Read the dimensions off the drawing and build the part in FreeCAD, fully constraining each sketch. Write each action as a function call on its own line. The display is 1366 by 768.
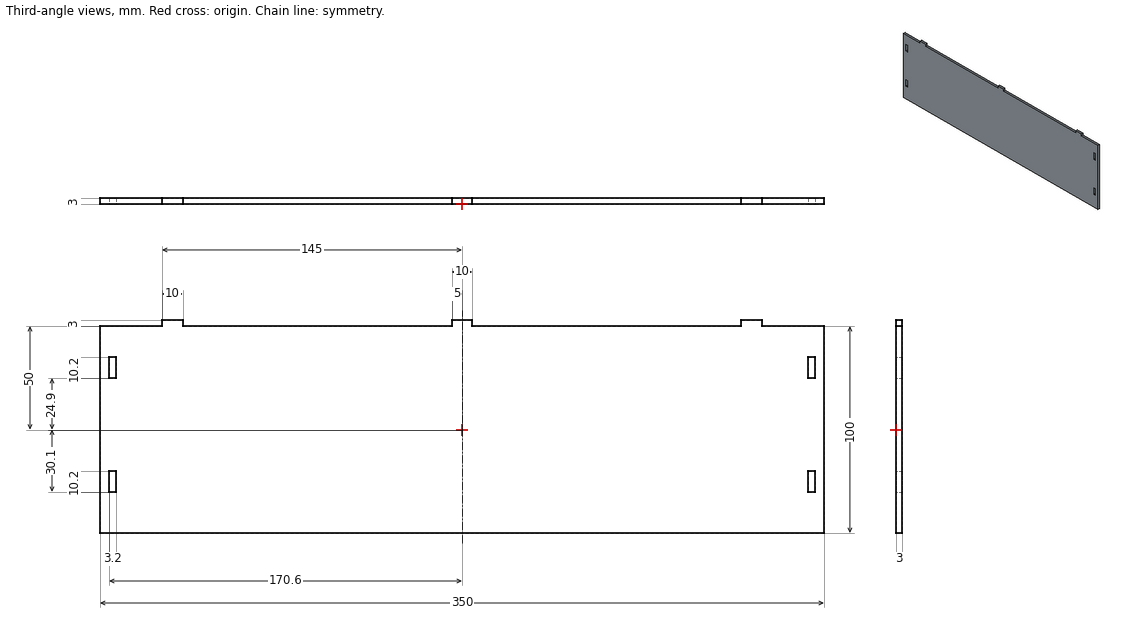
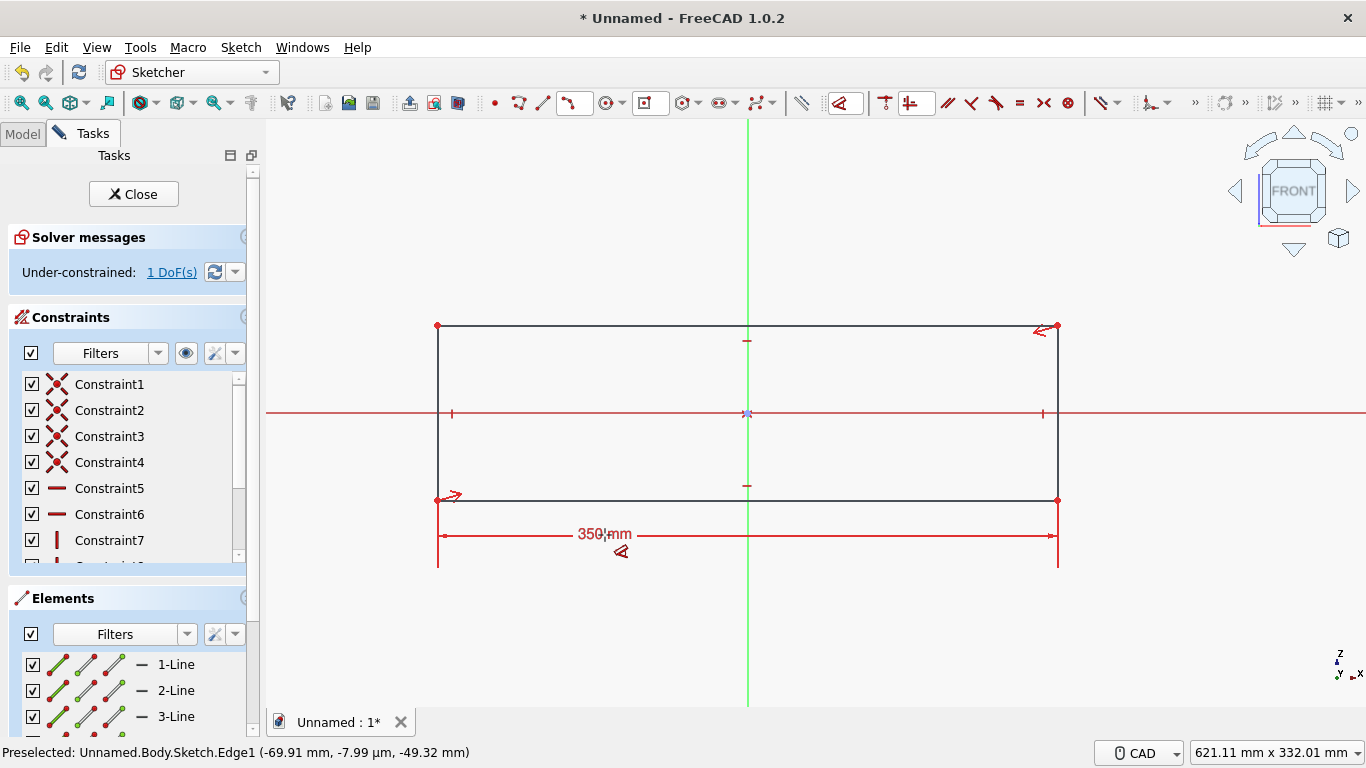
click(1058, 448)
click(1092, 373)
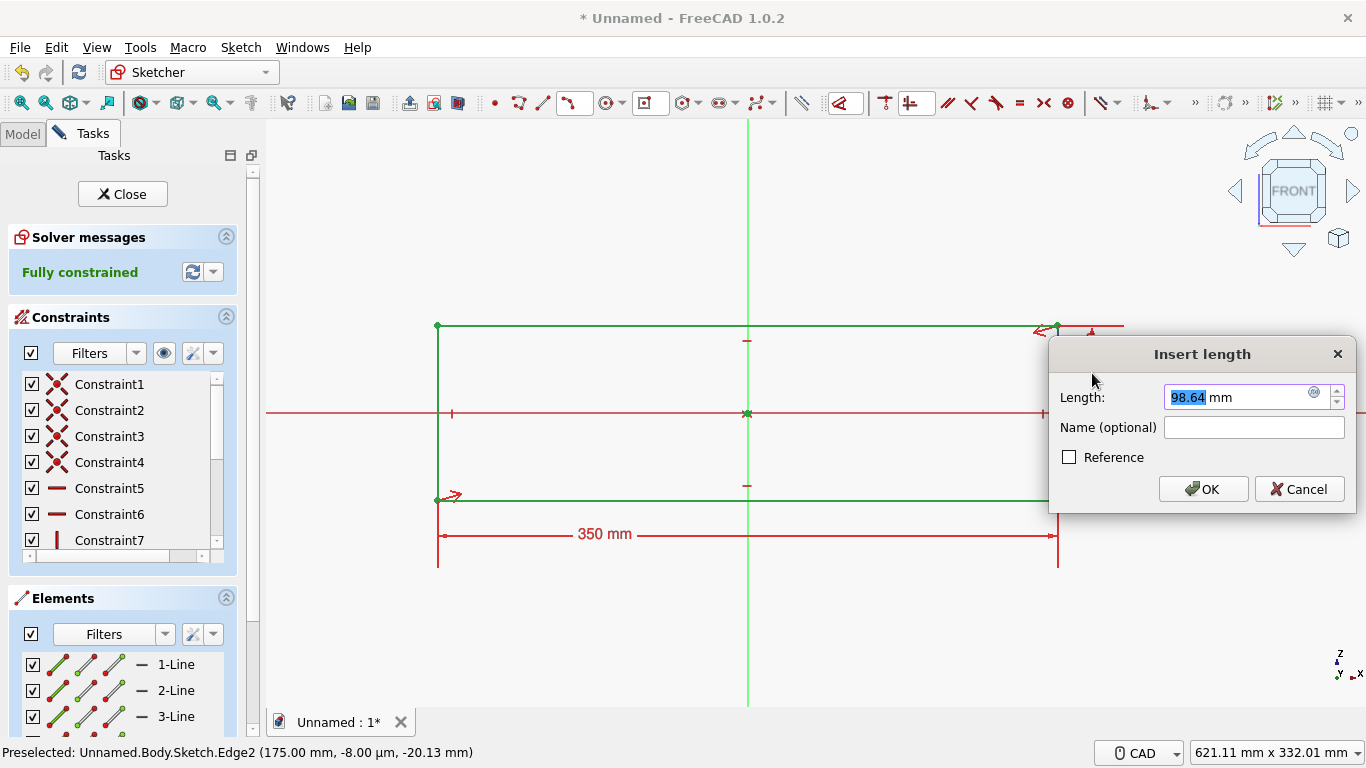
text(100)
key(Return)
key(Escape)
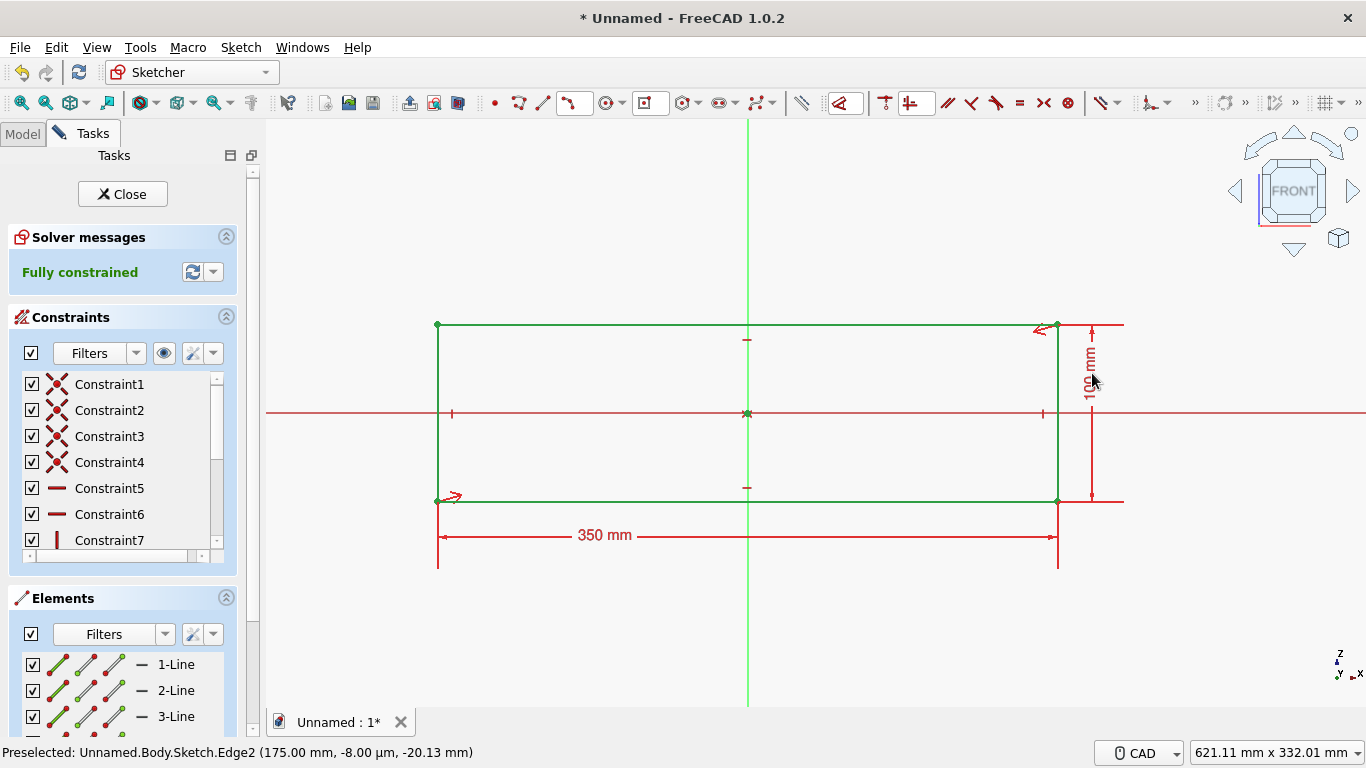
click(123, 194)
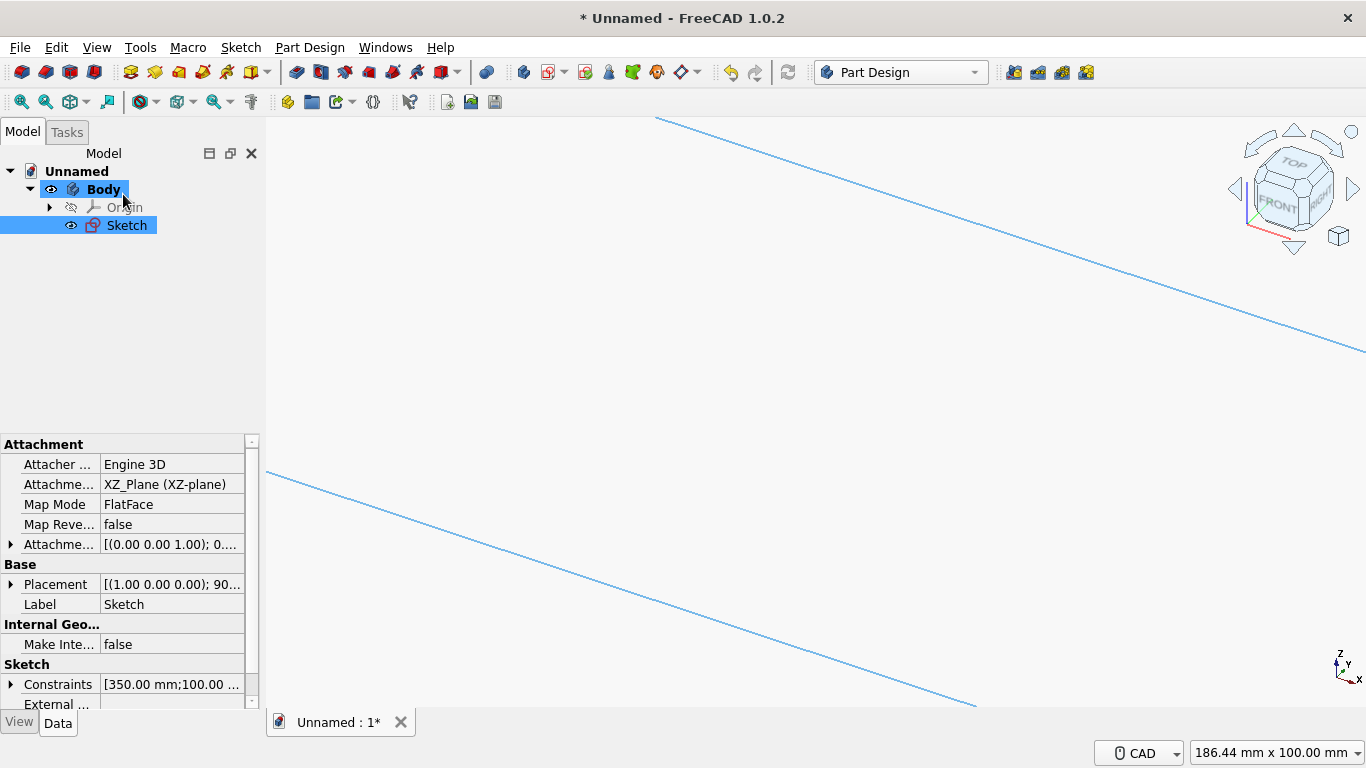
click(132, 72)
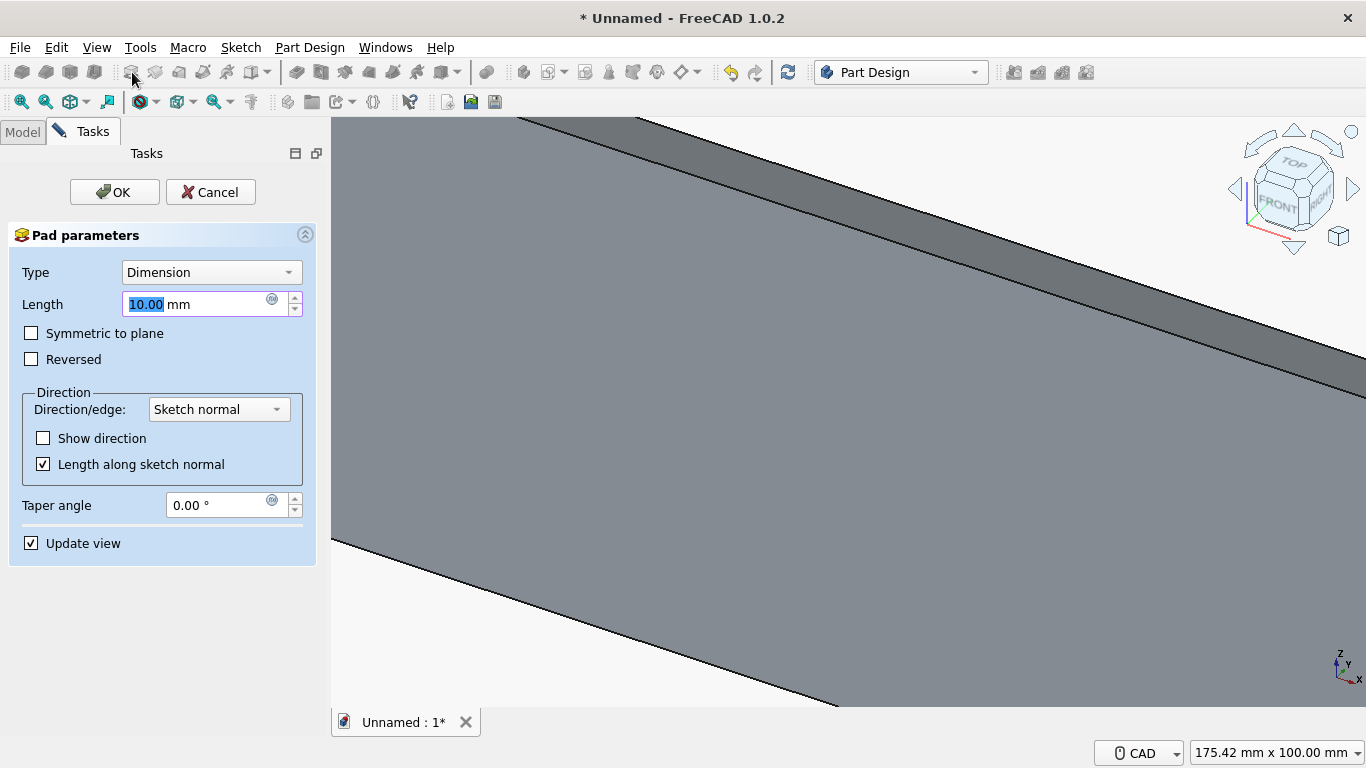
text(3)
key(Tab)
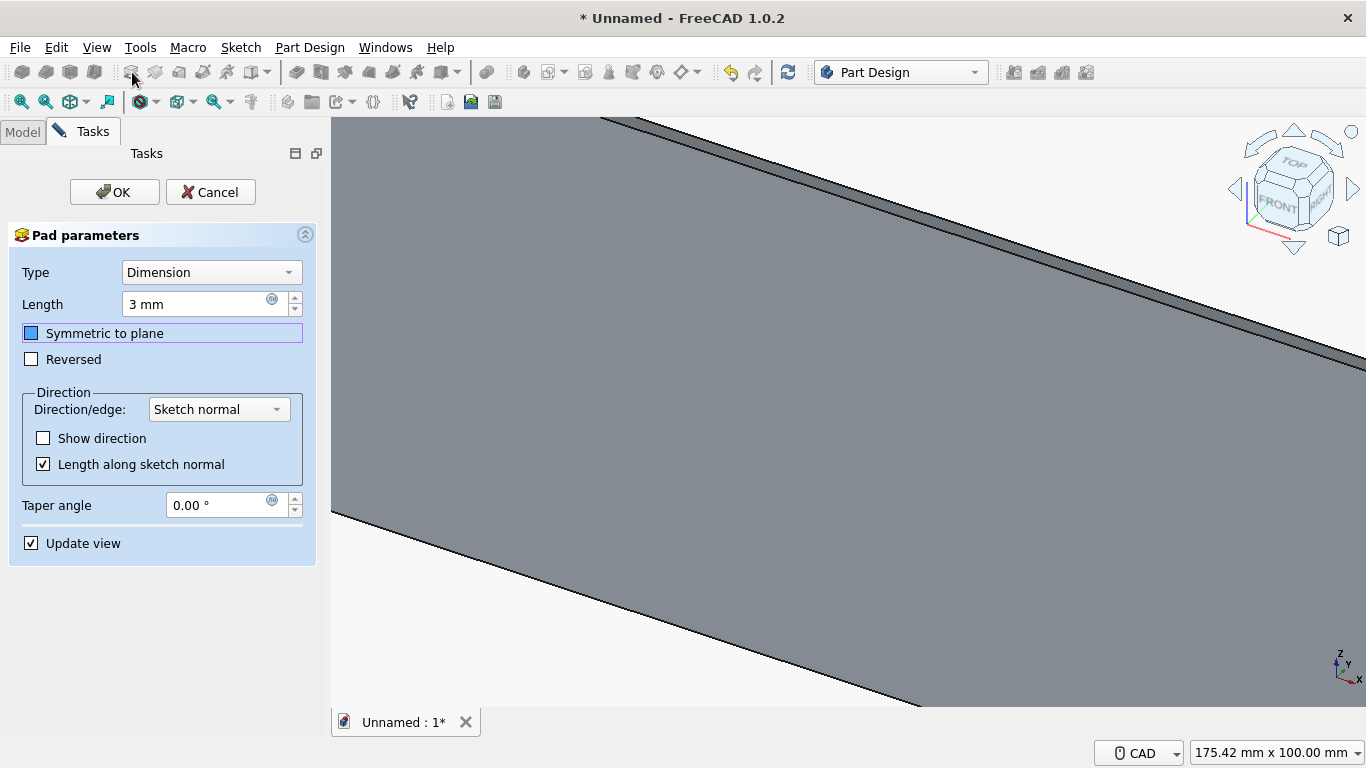
click(30, 359)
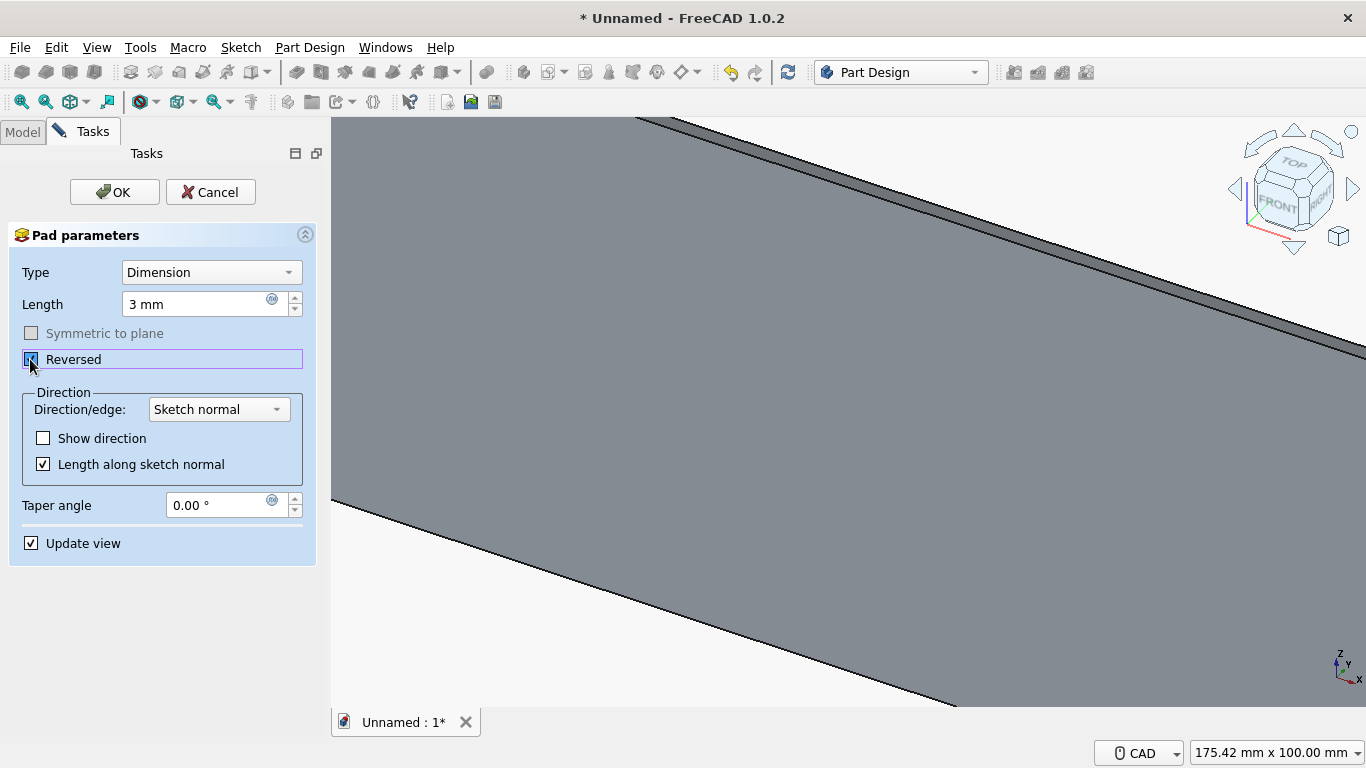
click(115, 192)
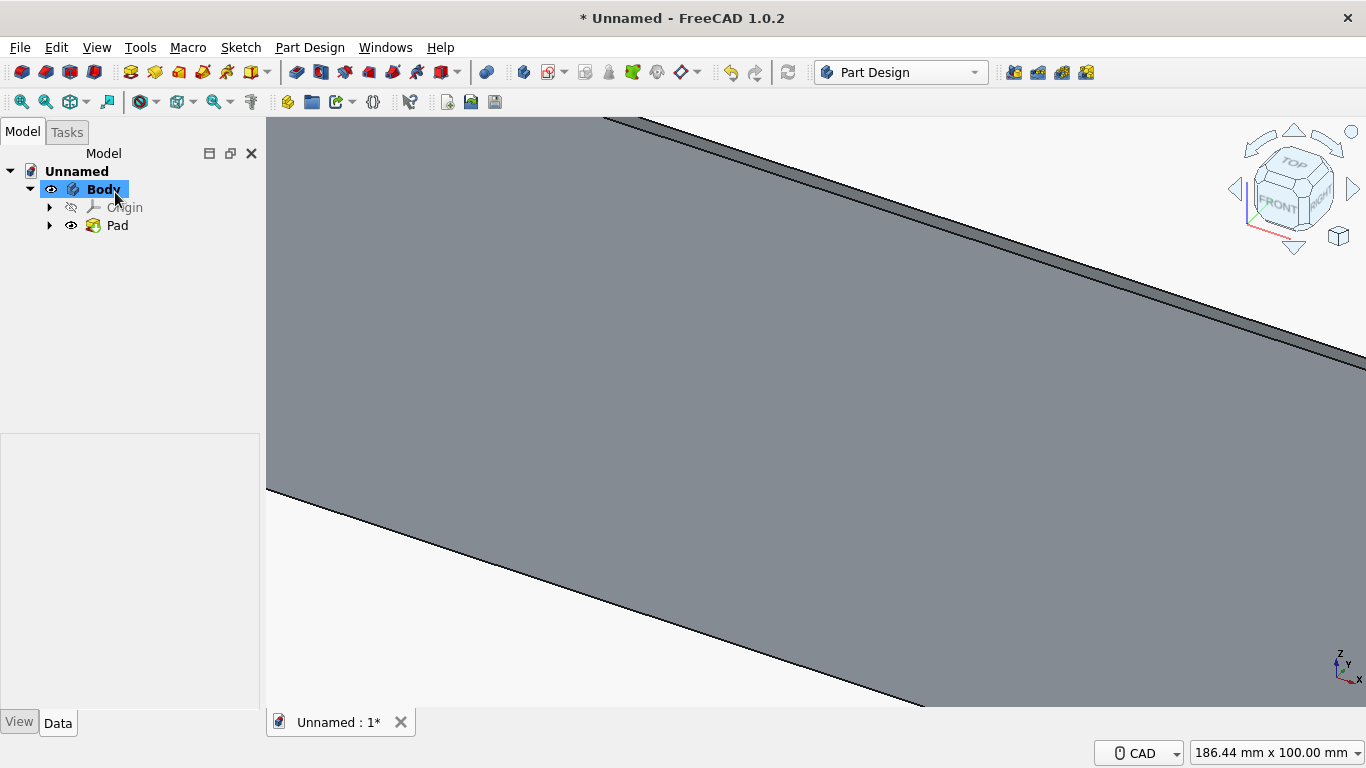
key(v)
key(f)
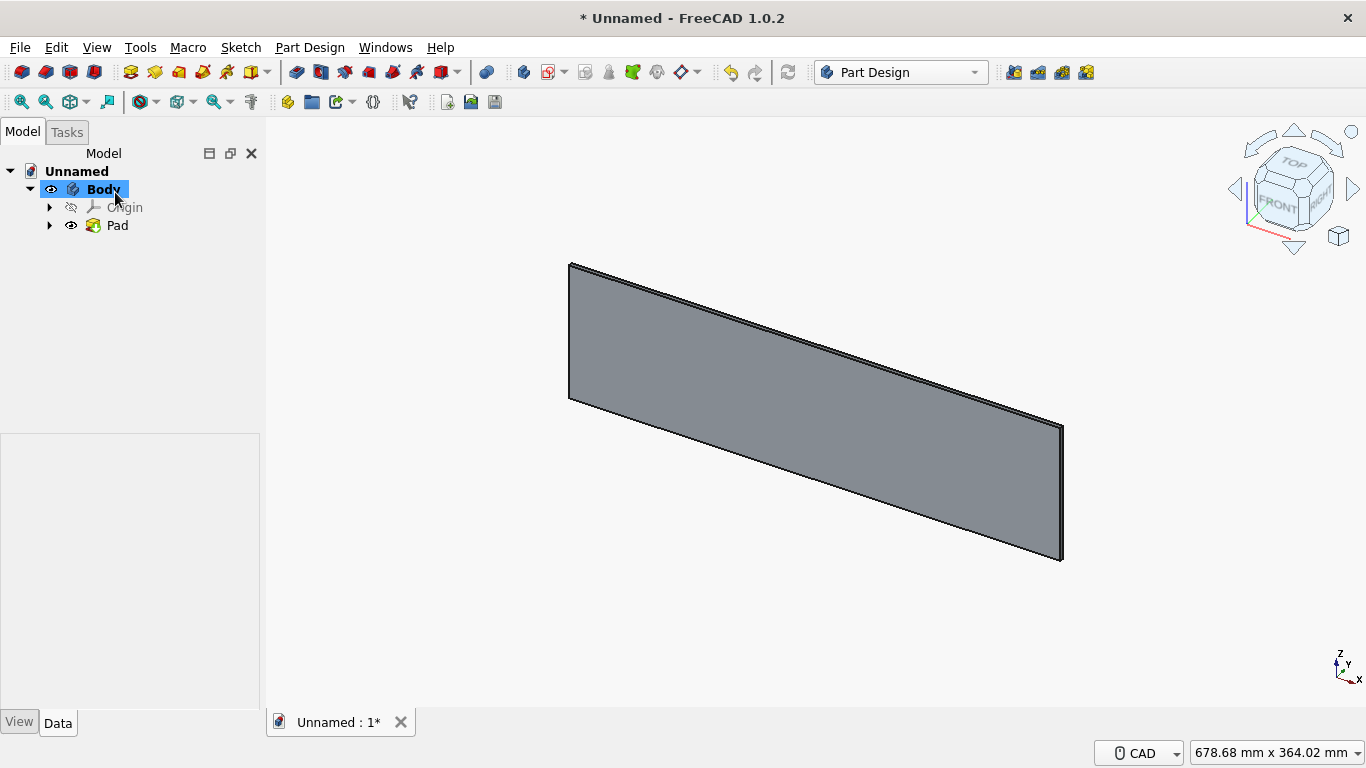
key(4)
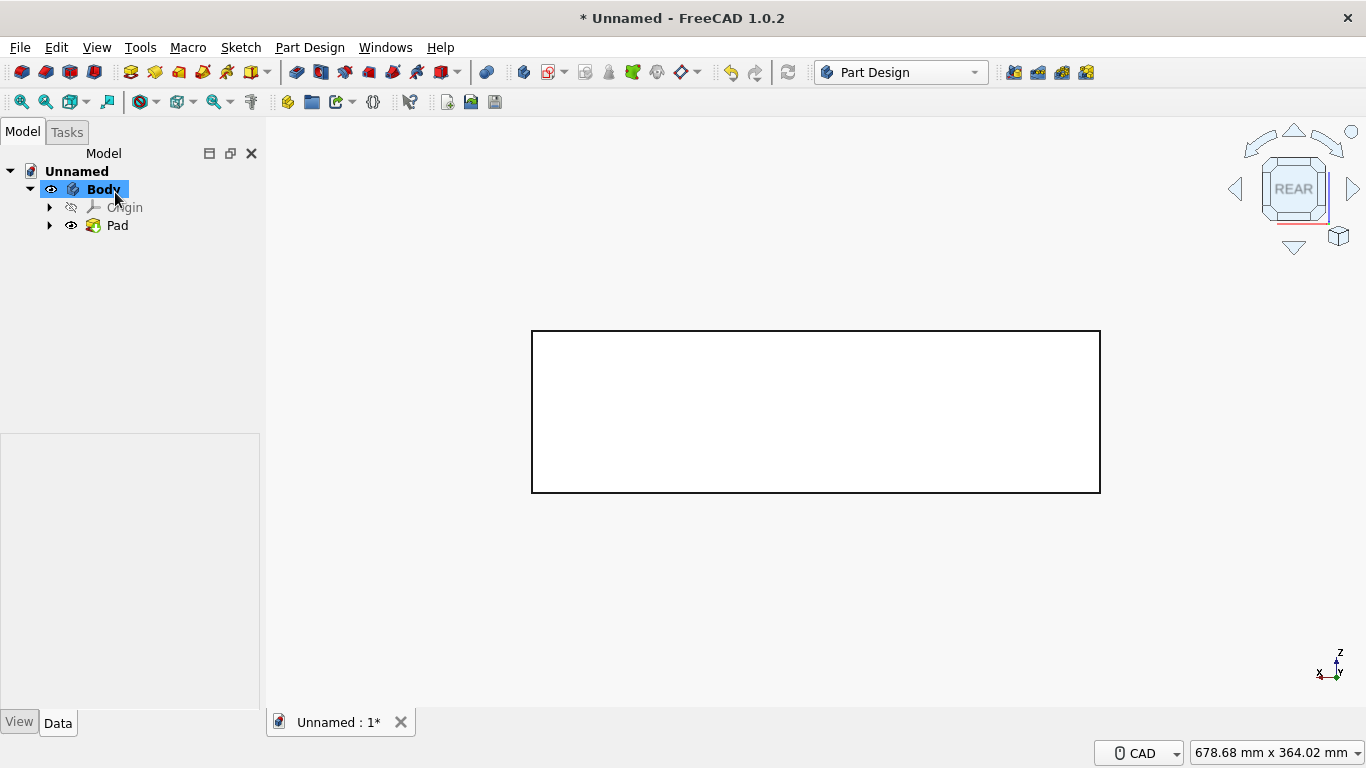
click(654, 411)